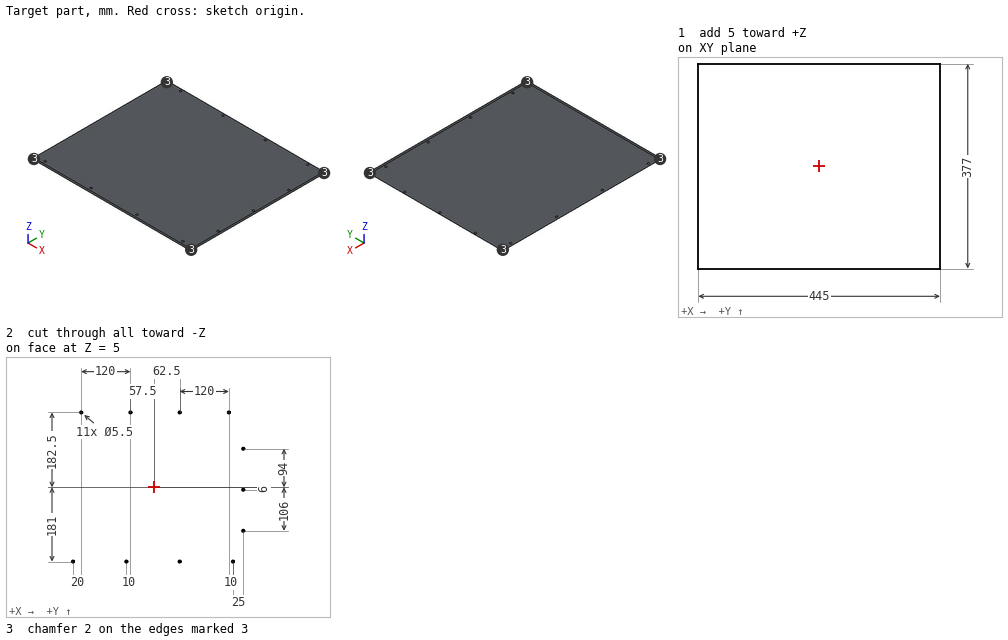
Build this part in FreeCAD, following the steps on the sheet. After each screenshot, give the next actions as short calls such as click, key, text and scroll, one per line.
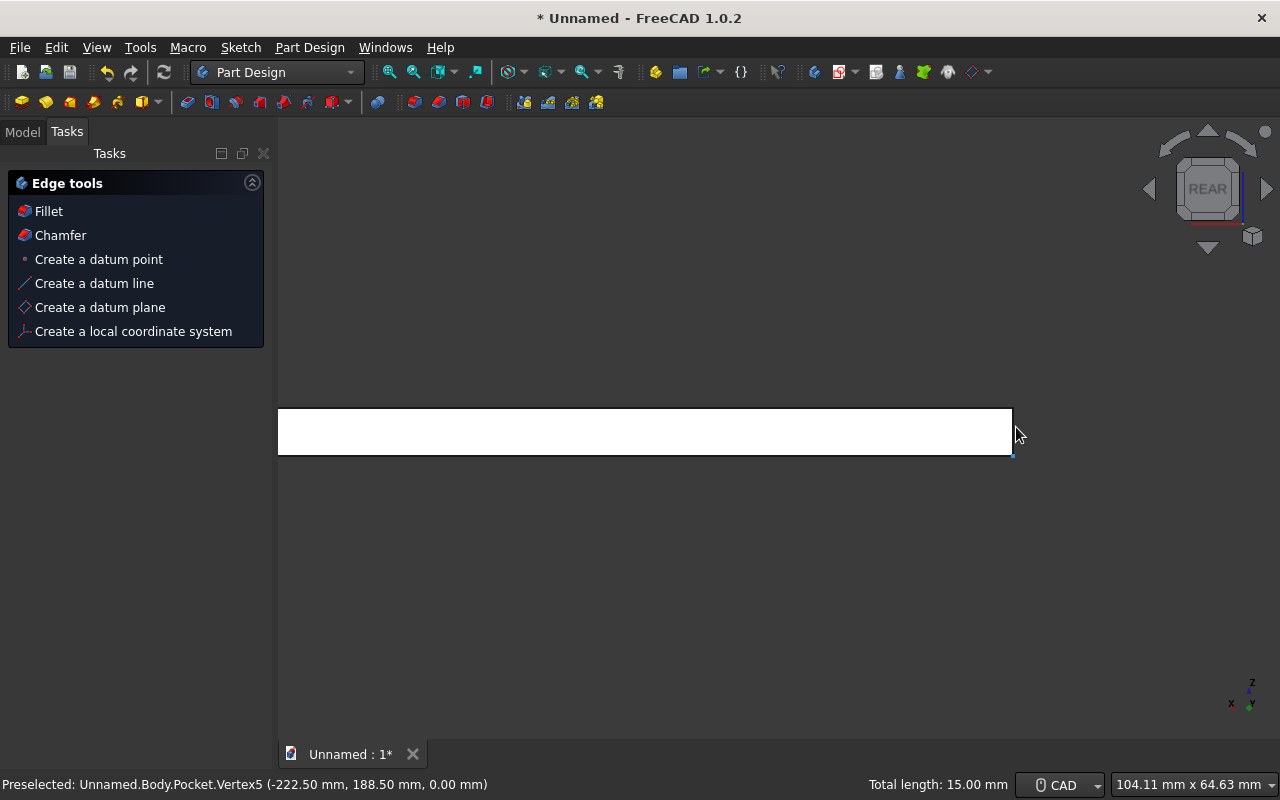
click(1013, 431, ctrl)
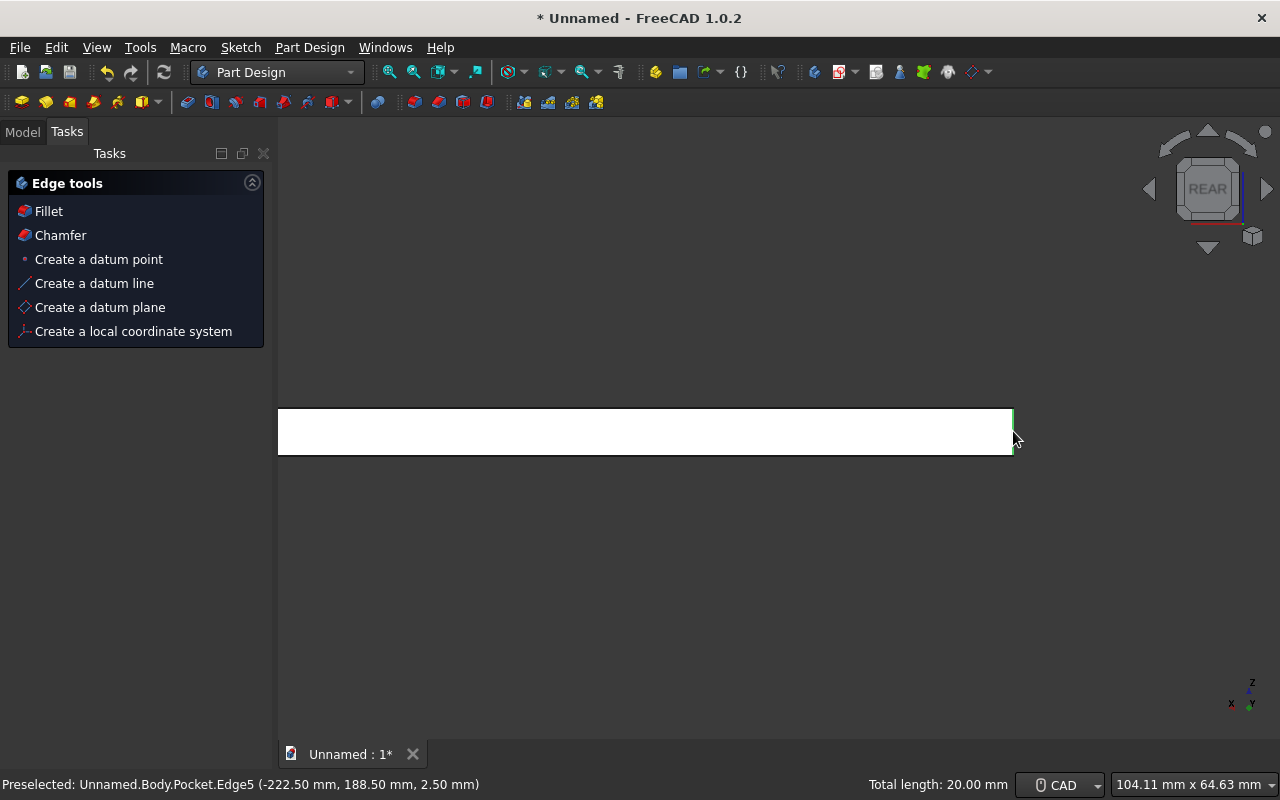
click(440, 102)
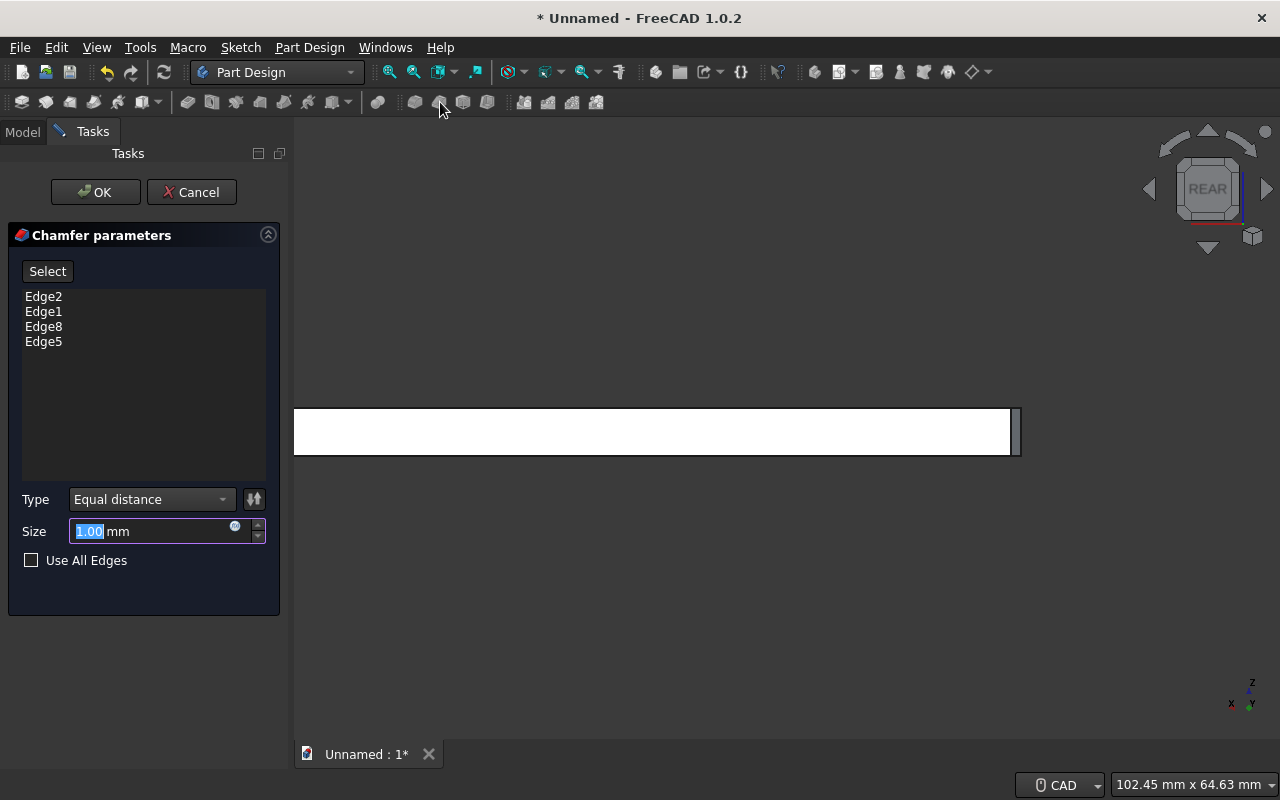
text(2)
key(Tab)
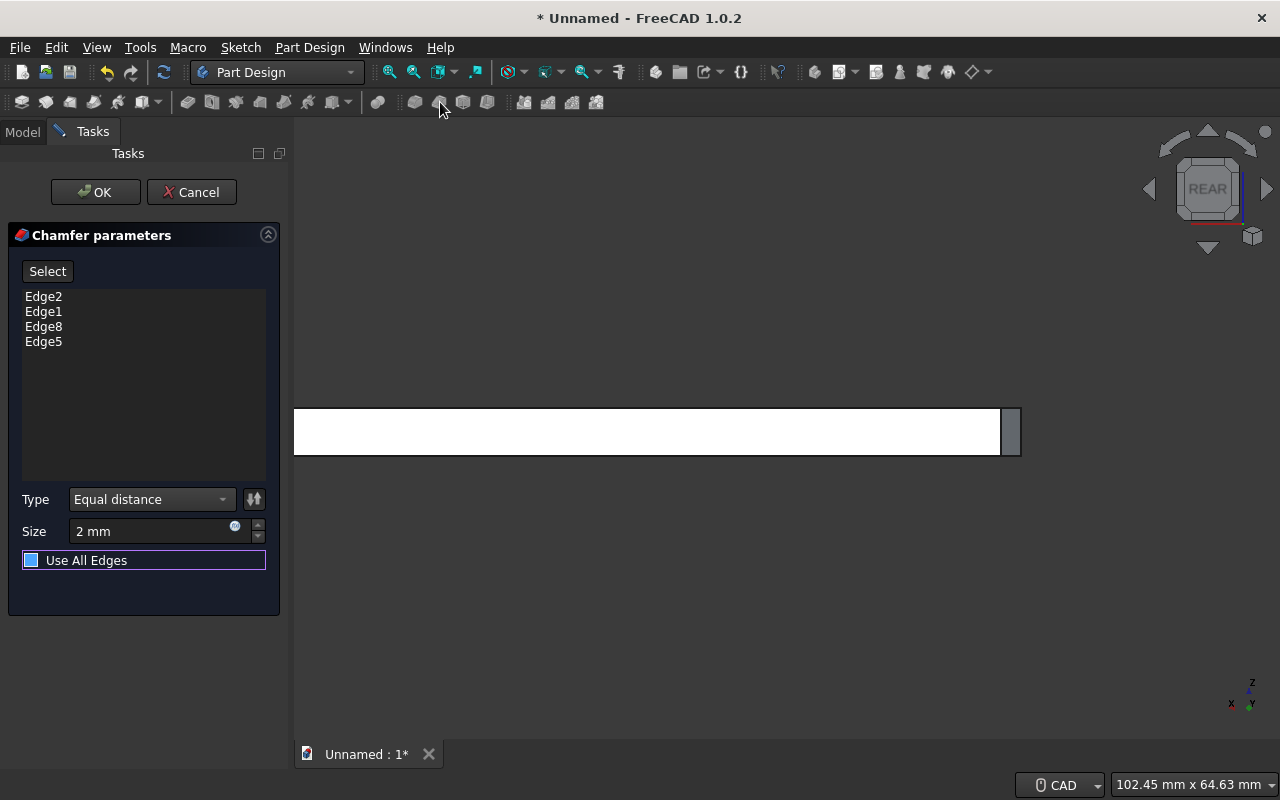
click(96, 192)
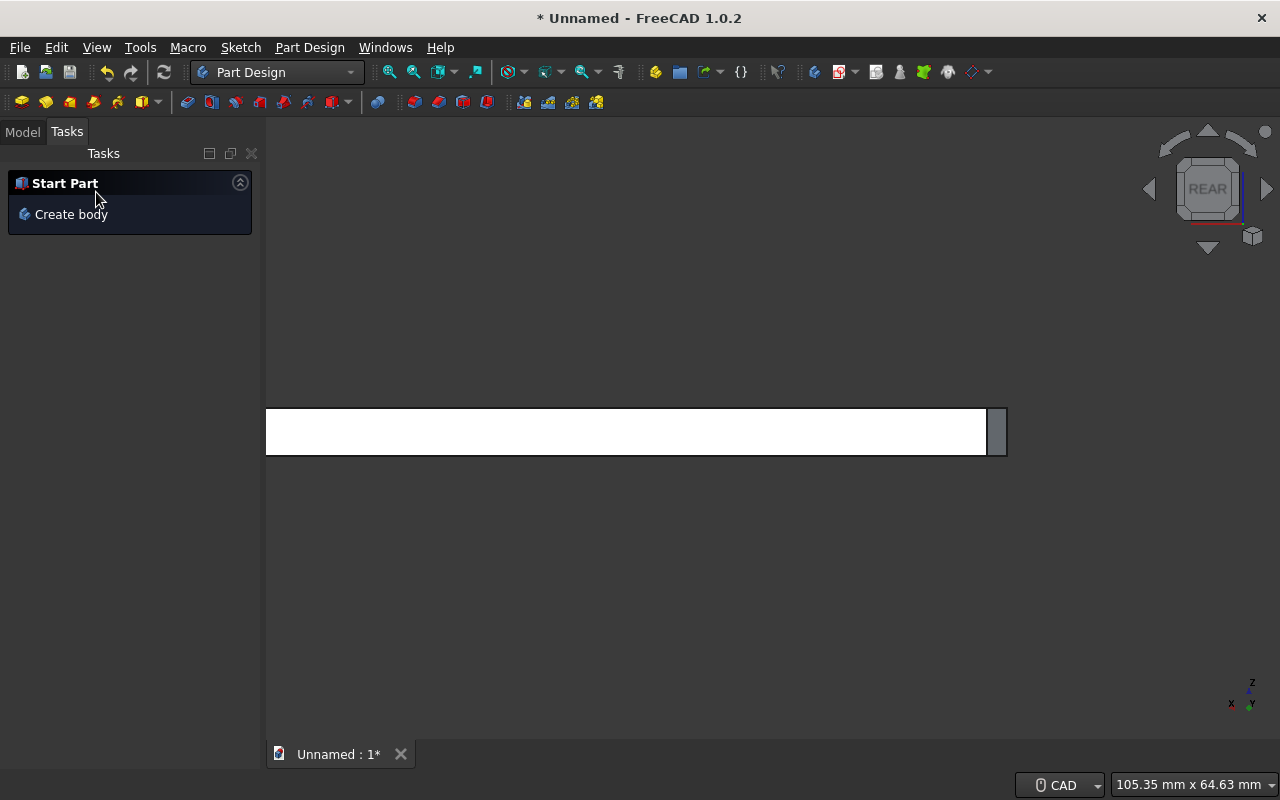
key(0)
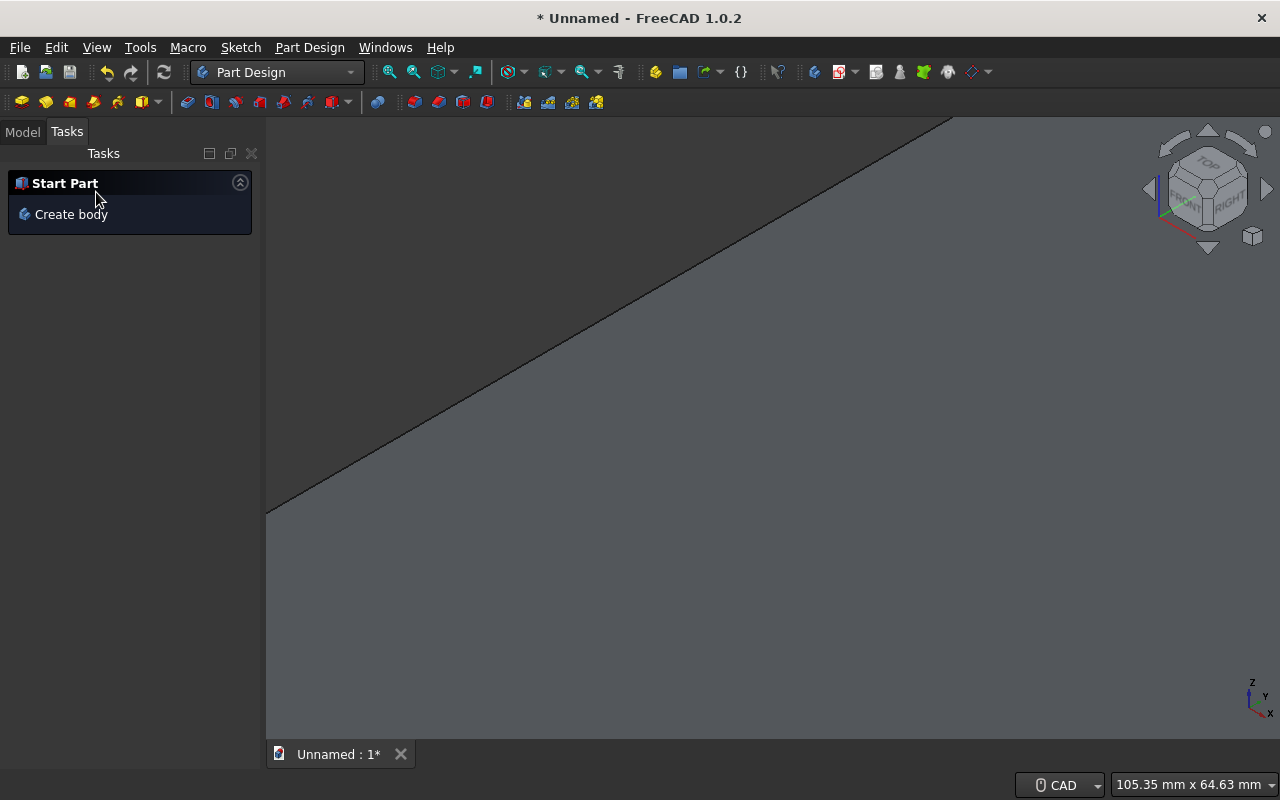
click(390, 72)